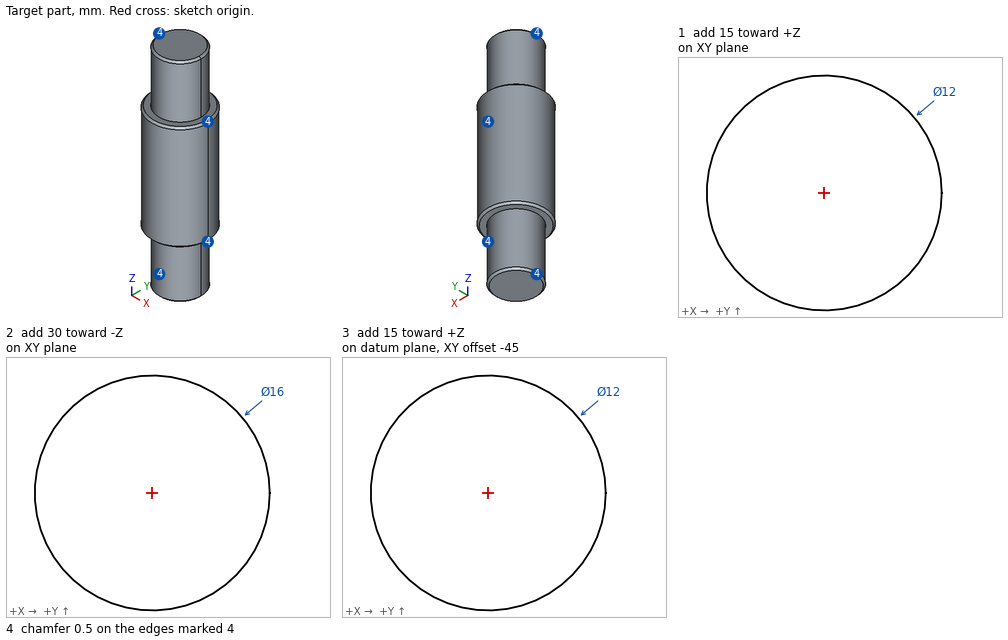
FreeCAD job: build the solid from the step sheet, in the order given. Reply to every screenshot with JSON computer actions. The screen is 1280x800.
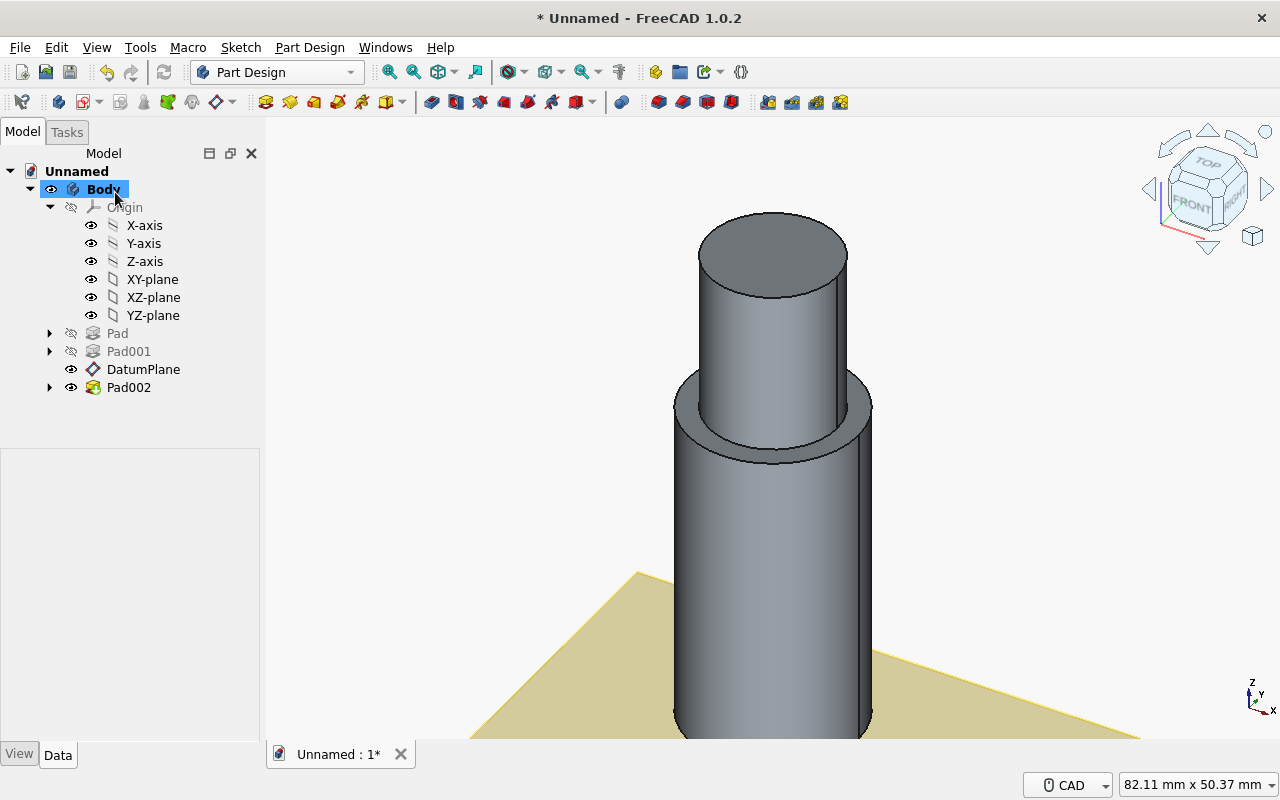
{"action": "left_click", "coordinate": [116, 369]}
{"action": "key", "text": "space"}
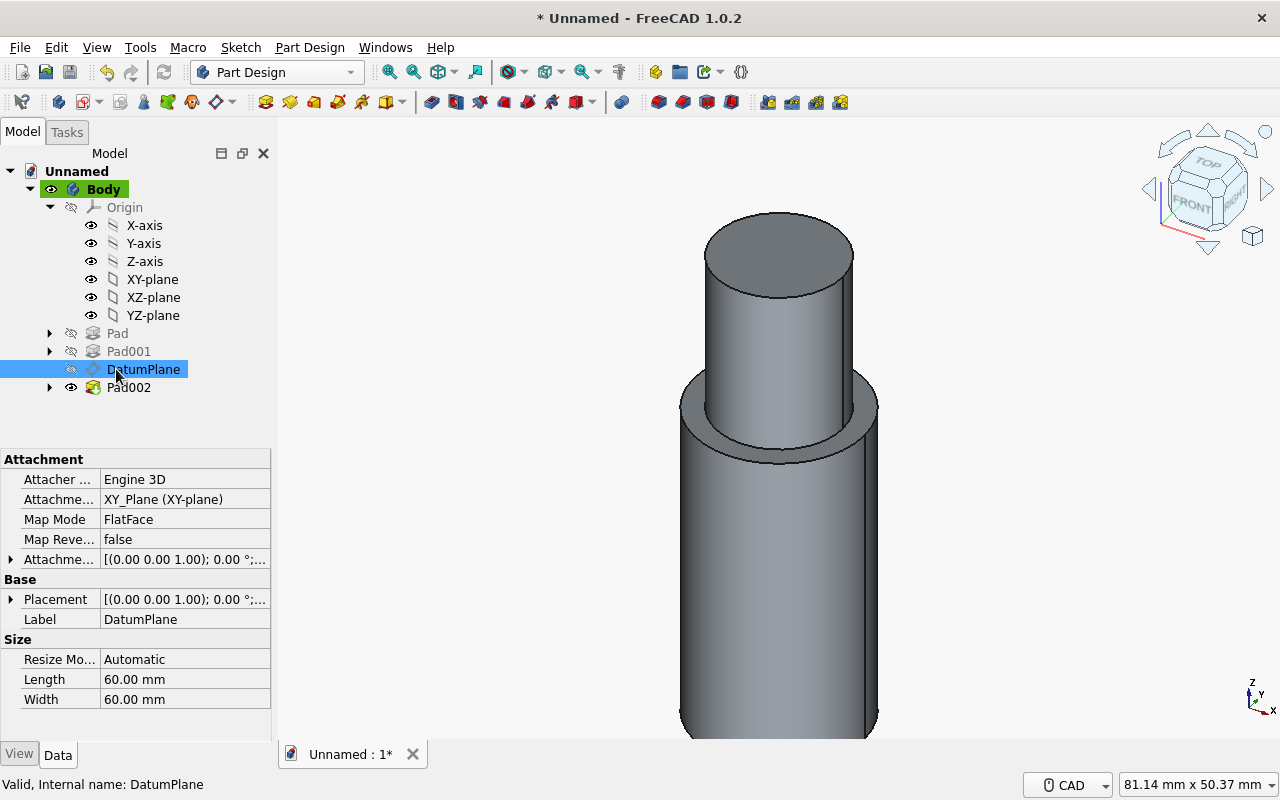
{"action": "left_click", "coordinate": [390, 72]}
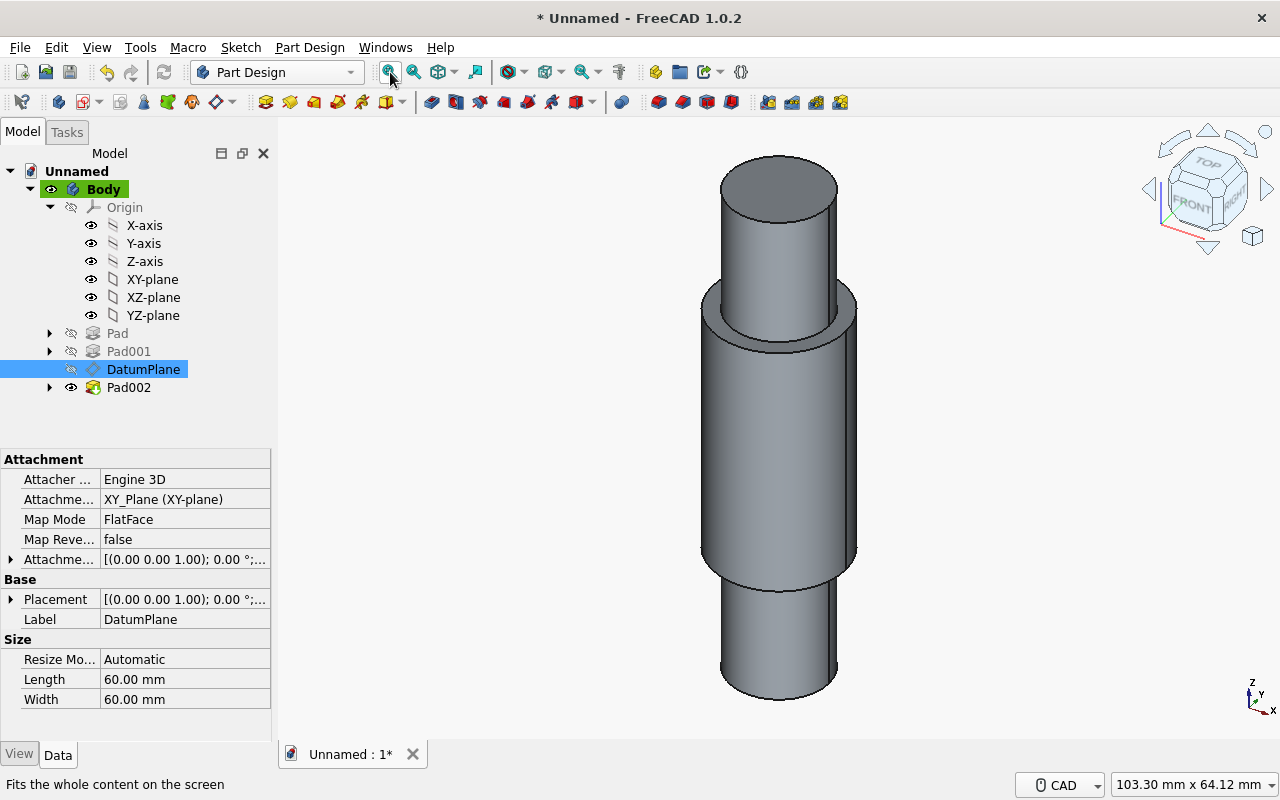
{"action": "left_click", "coordinate": [721, 192]}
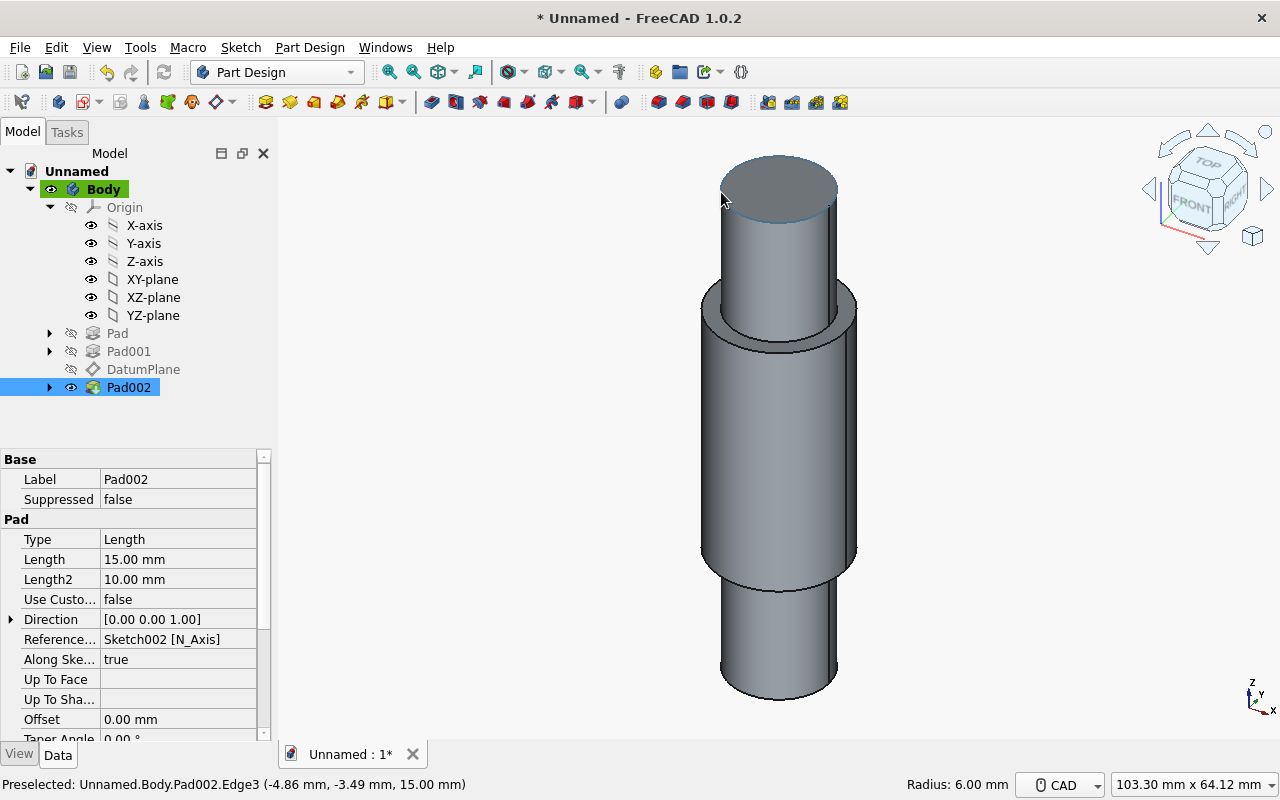
{"action": "left_click", "coordinate": [702, 312], "text": "ctrl"}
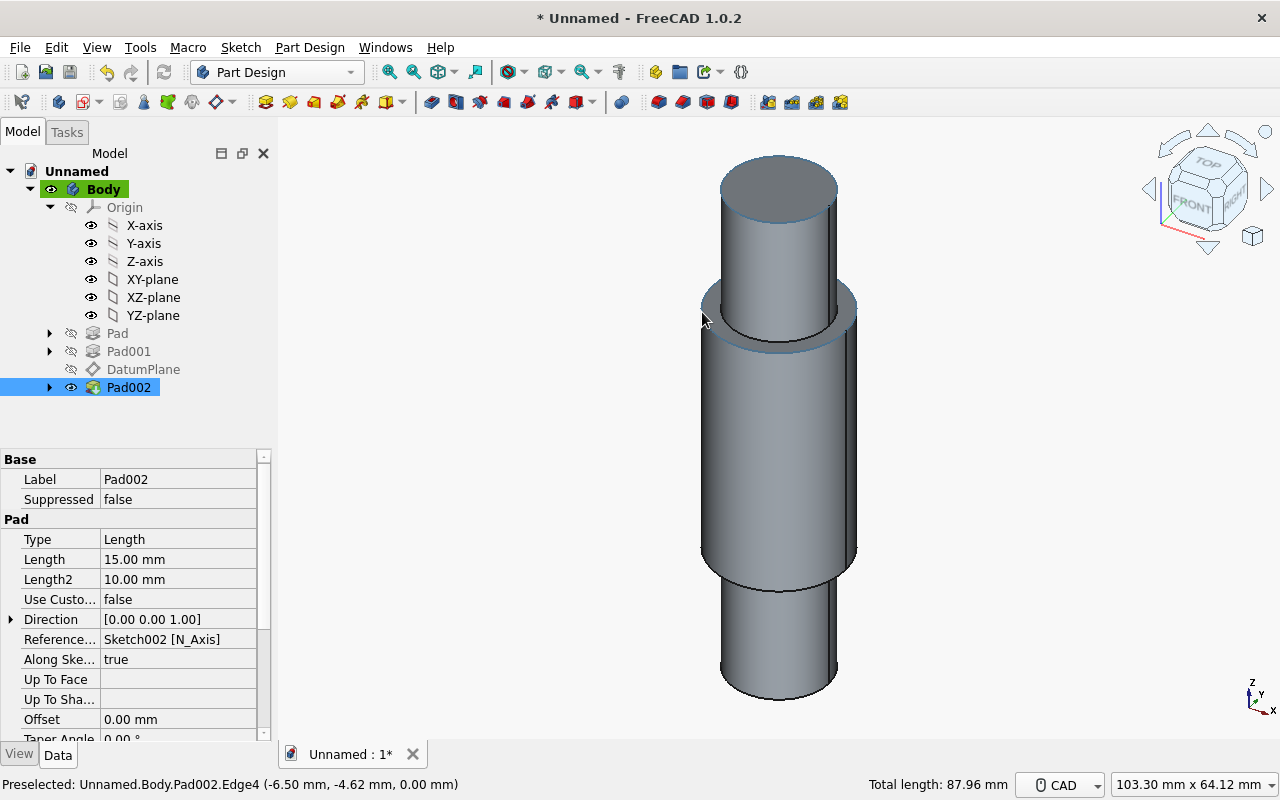
{"action": "key", "text": "0"}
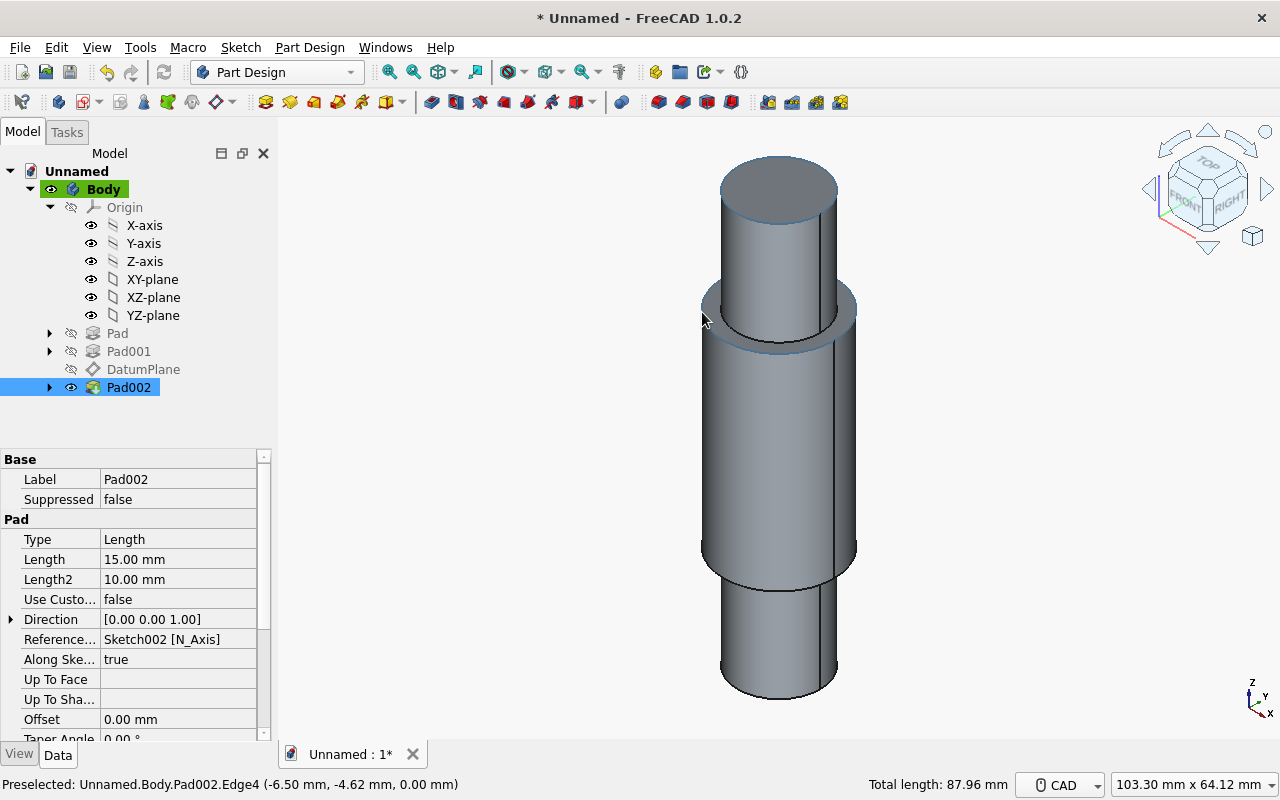
{"action": "key", "text": "2"}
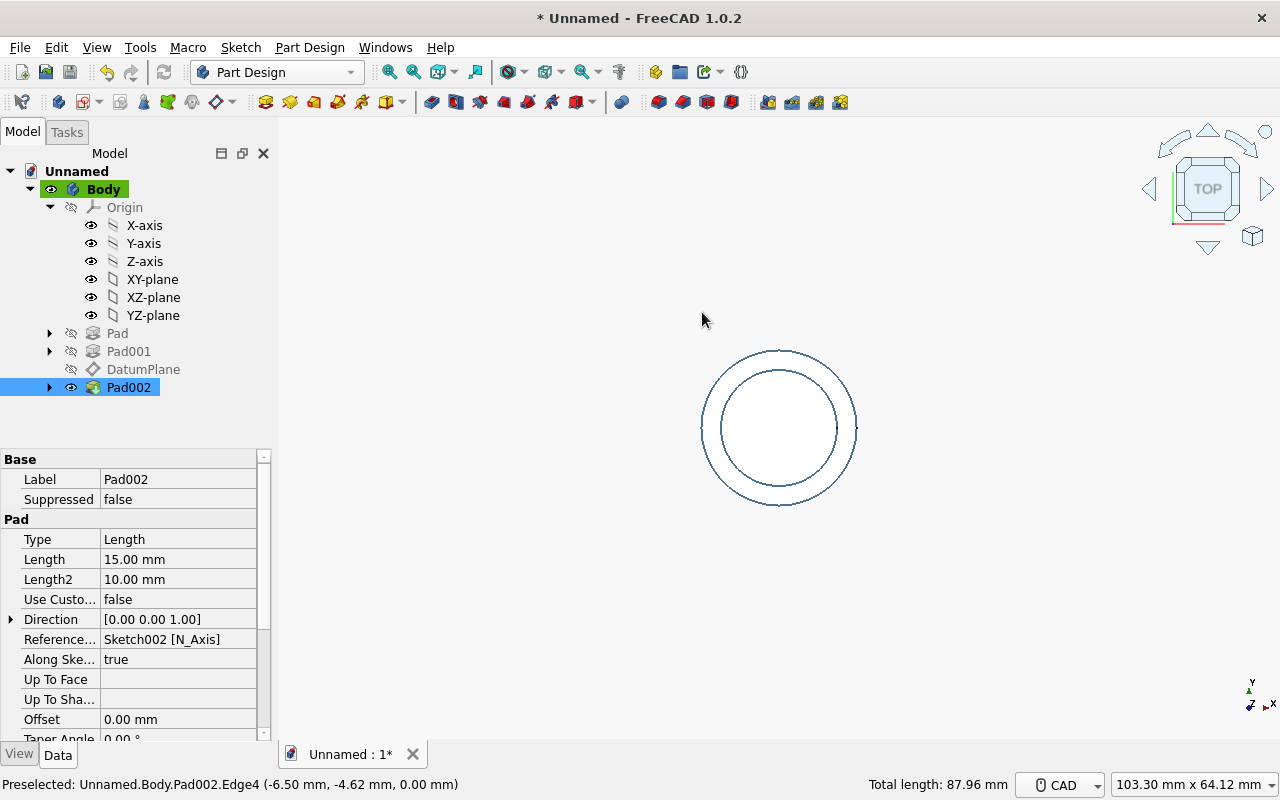
{"action": "left_click", "coordinate": [390, 72]}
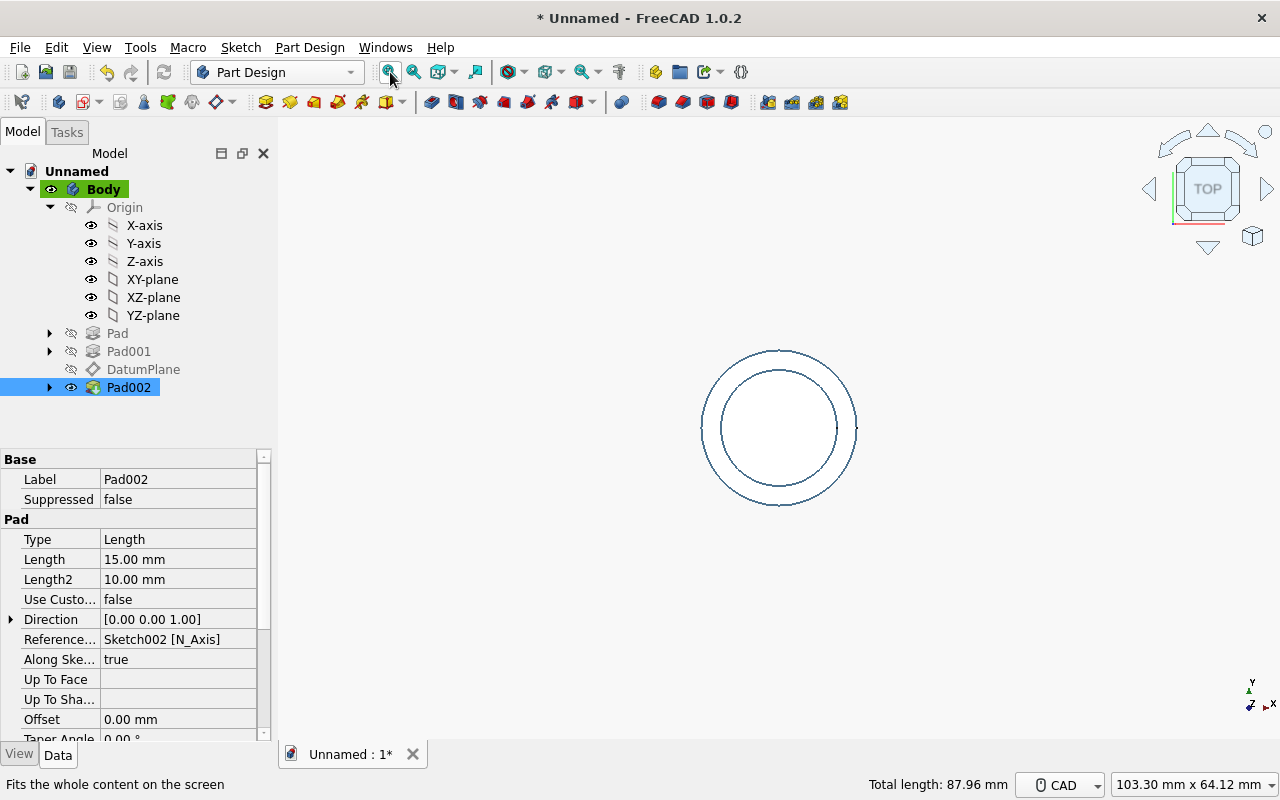
{"action": "key", "text": "1"}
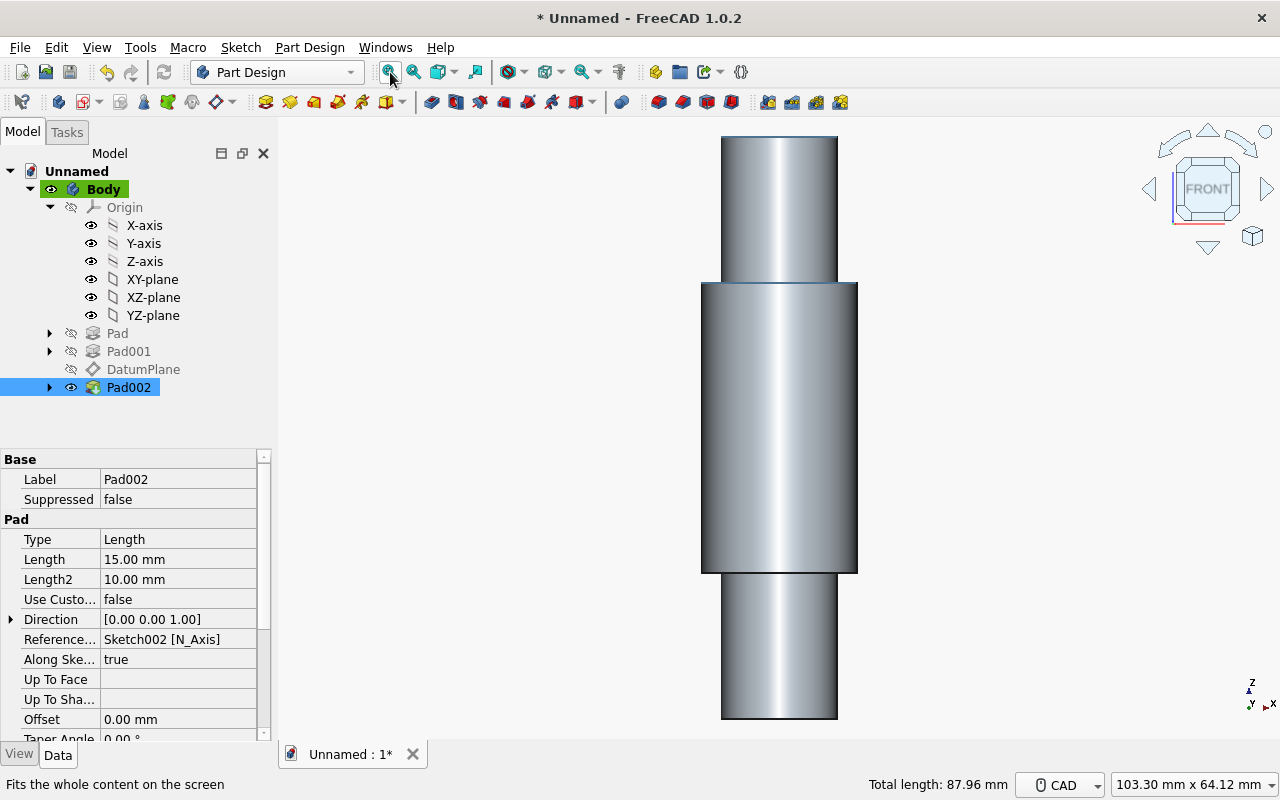
{"action": "left_click", "coordinate": [716, 572], "text": "ctrl"}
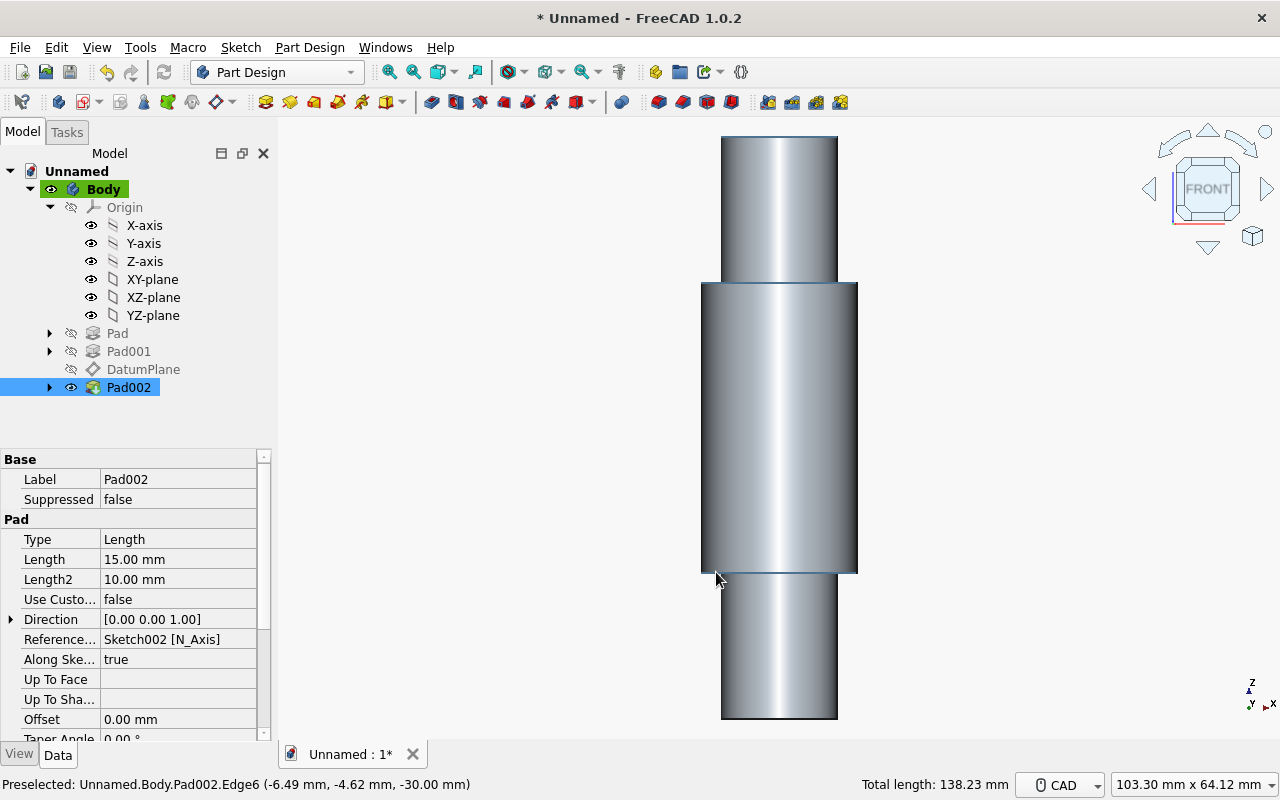
{"action": "key", "text": "3"}